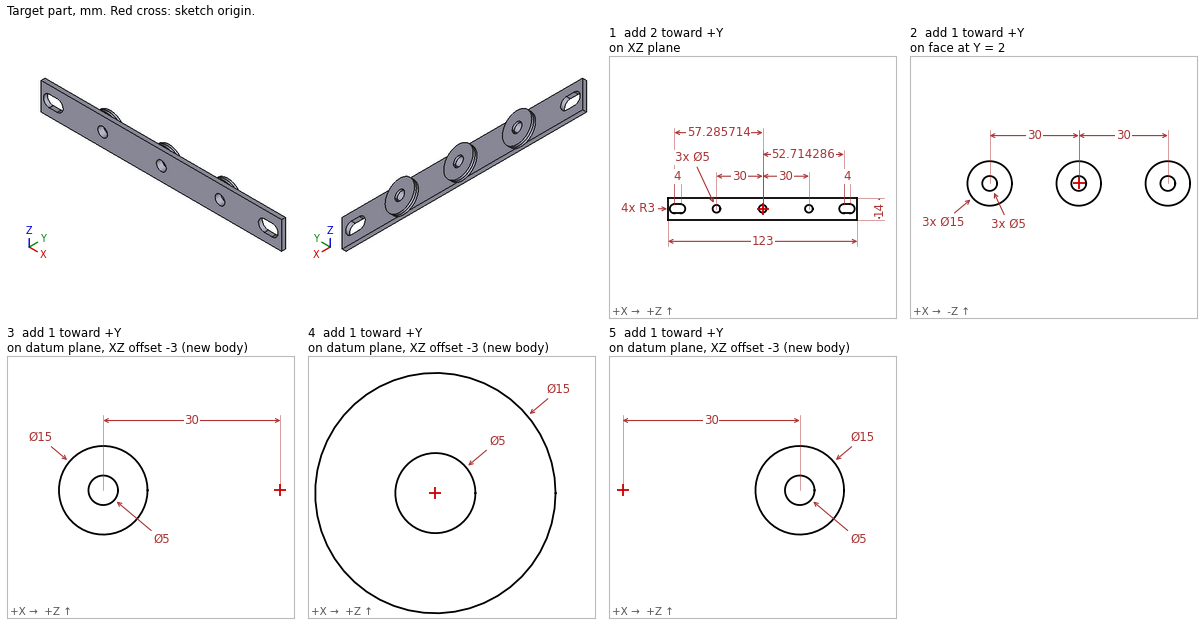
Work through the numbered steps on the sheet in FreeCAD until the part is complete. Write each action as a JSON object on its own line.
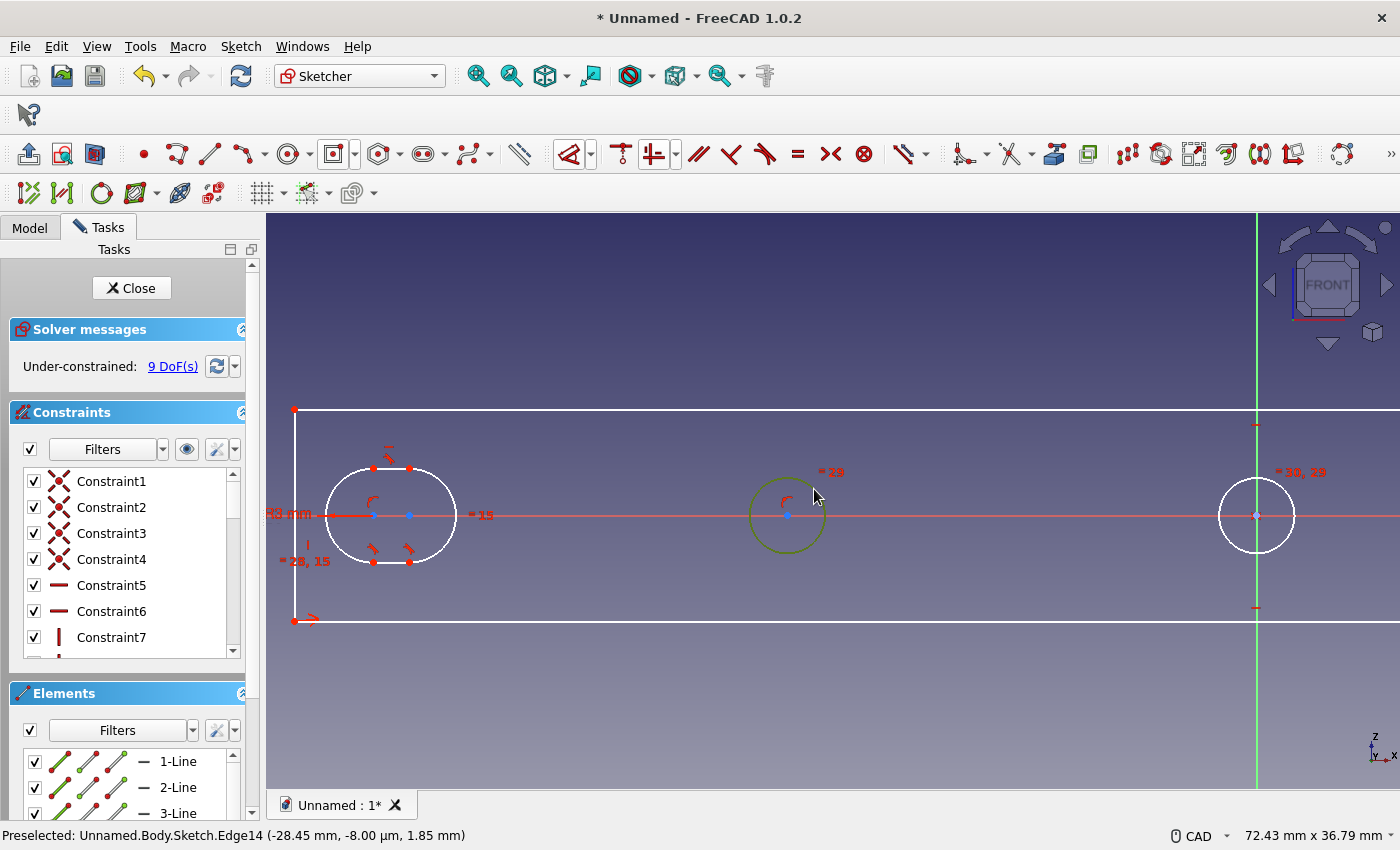
{"action": "left_click", "coordinate": [590, 154]}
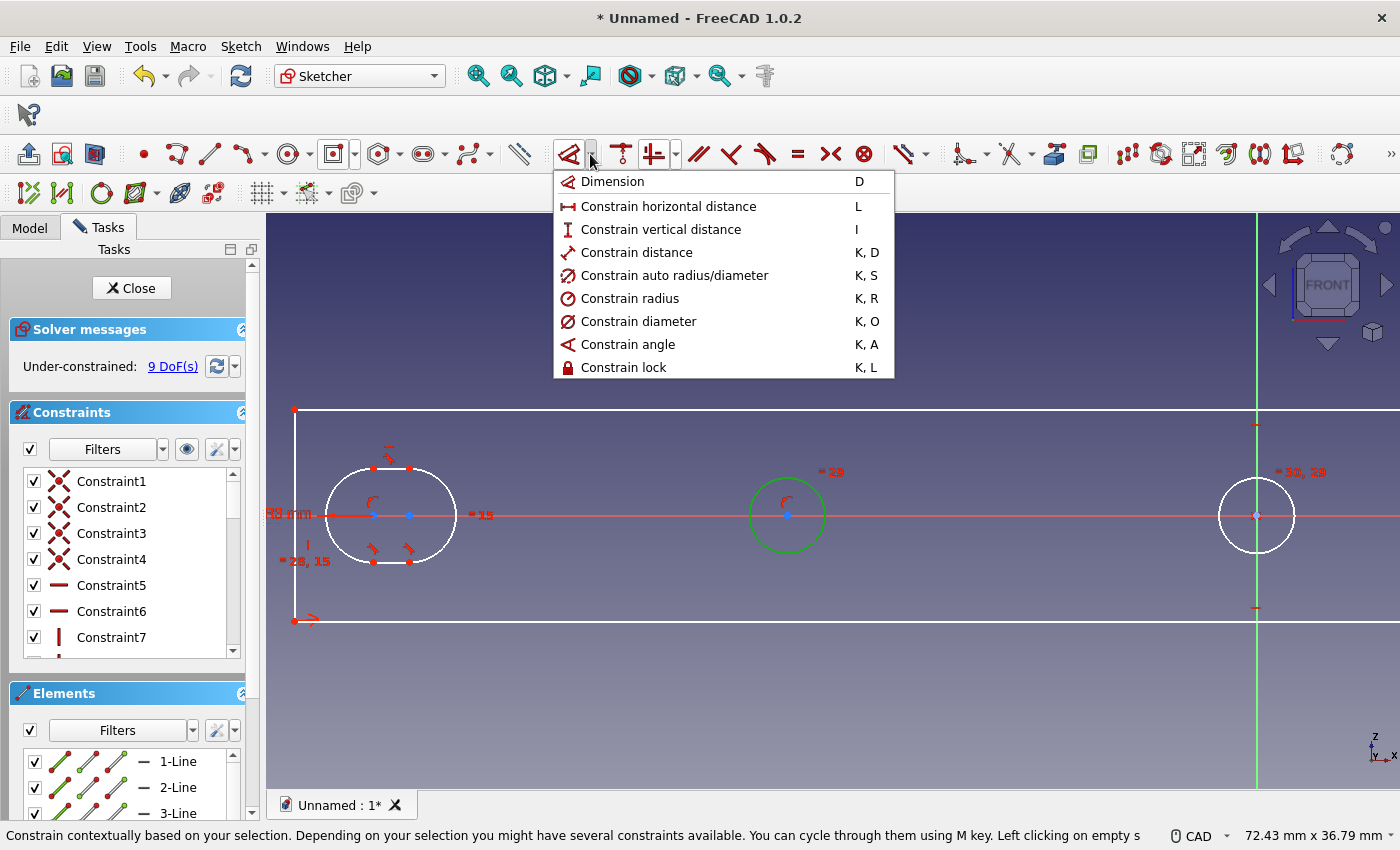
{"action": "left_click", "coordinate": [724, 322]}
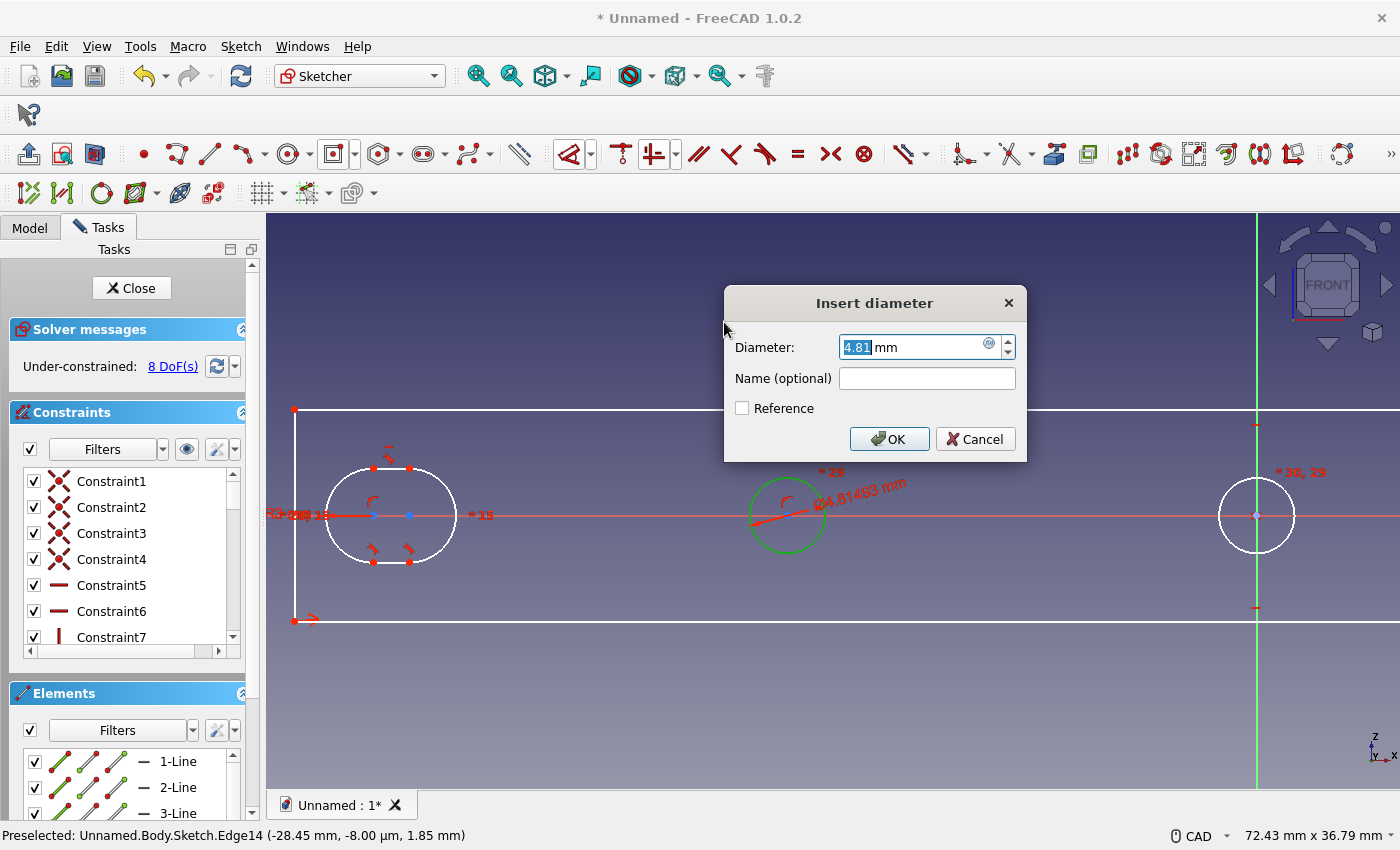
{"action": "type", "text": "5"}
{"action": "key", "text": "Return"}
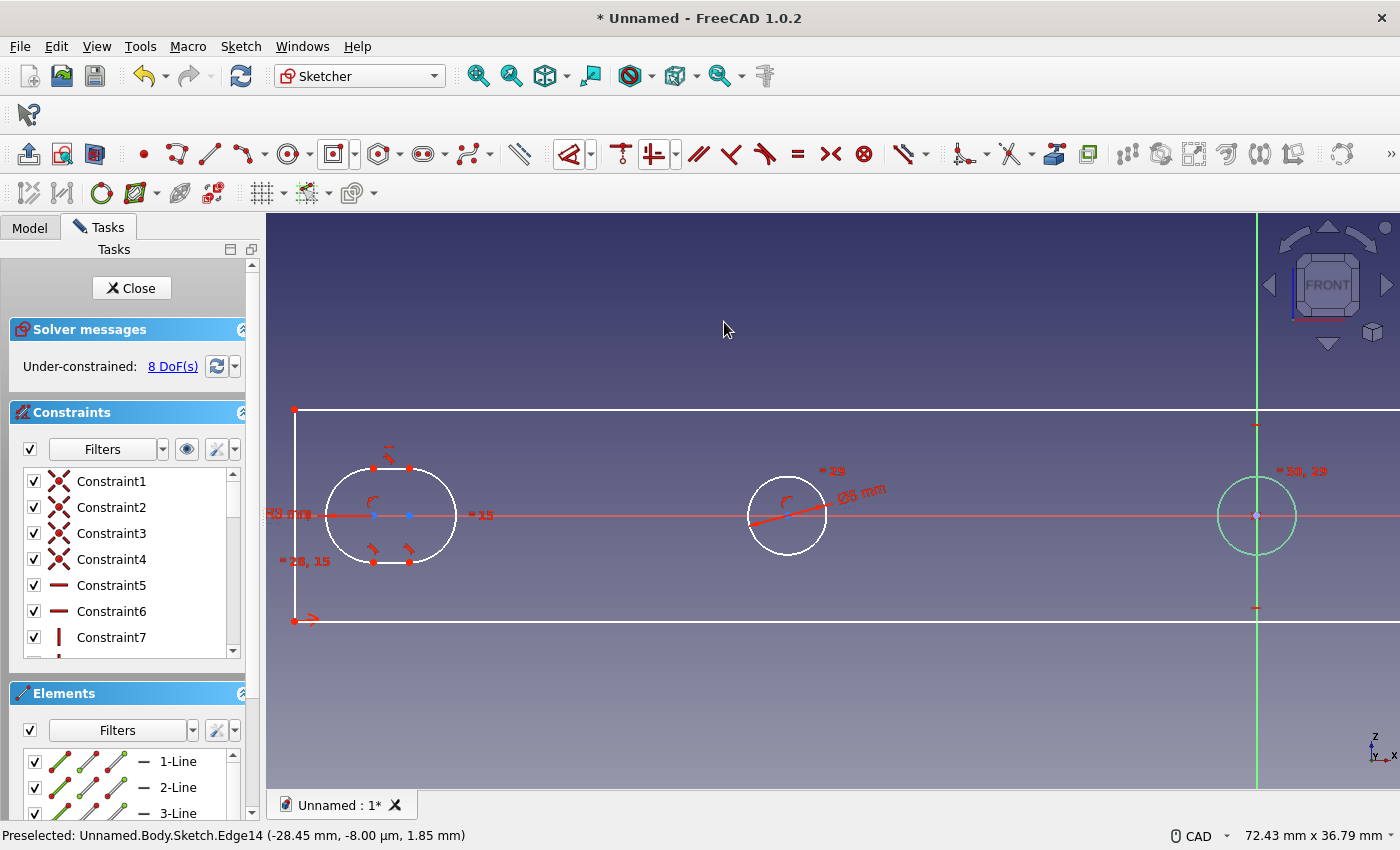
{"action": "scroll", "coordinate": [384, 469], "scroll_direction": "up", "scroll_amount": 2}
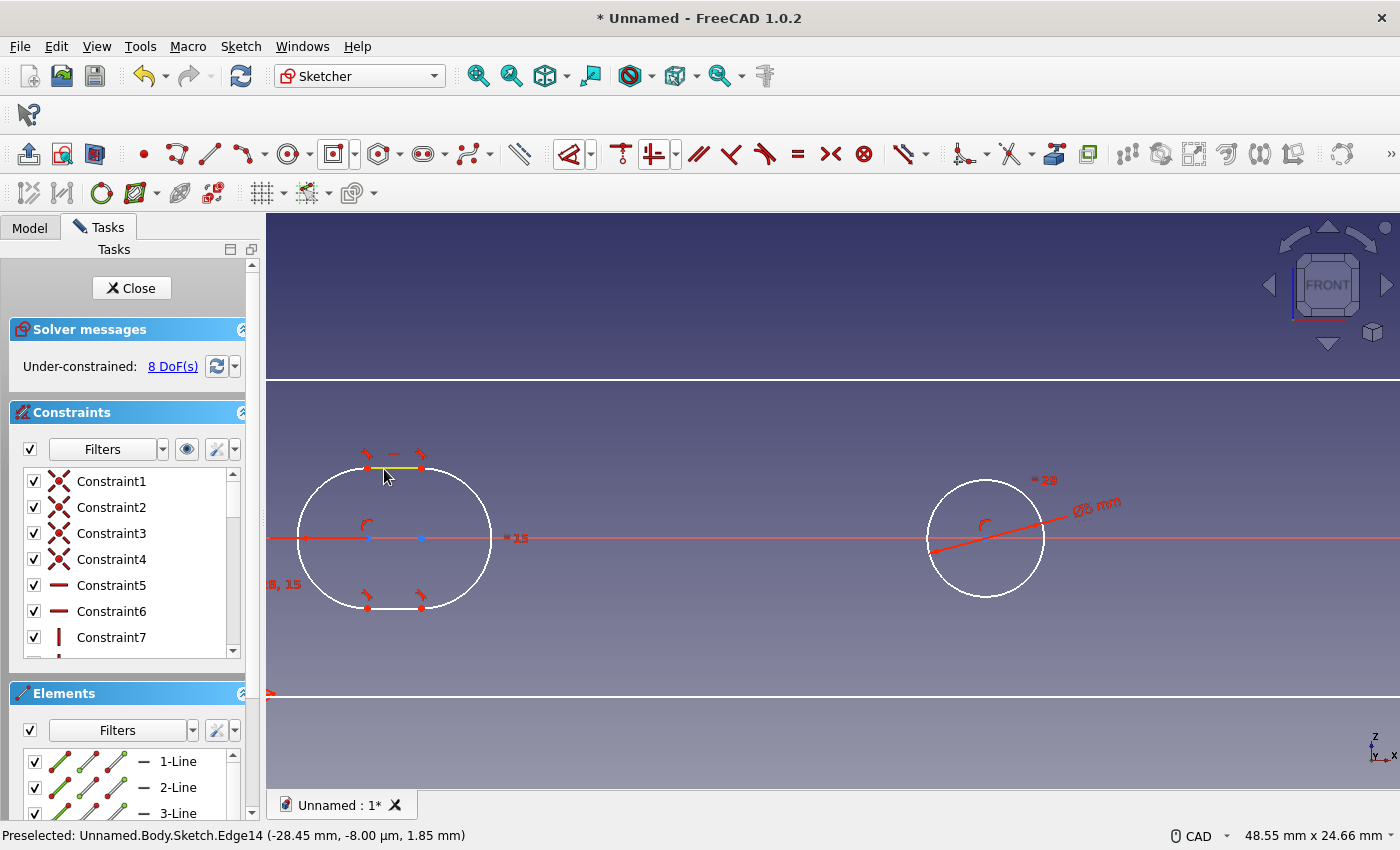
{"action": "left_click", "coordinate": [384, 468]}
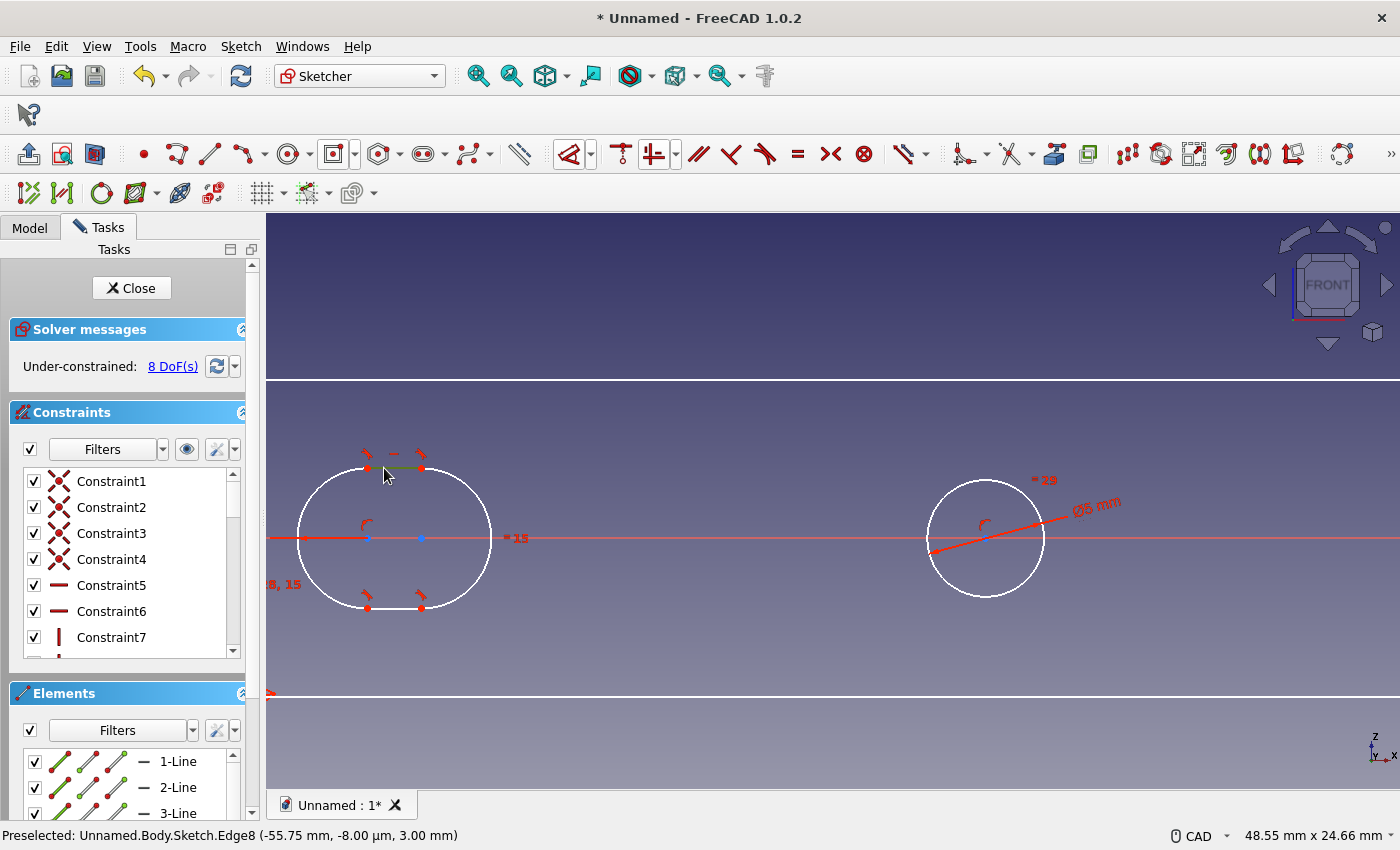
{"action": "key", "text": "l"}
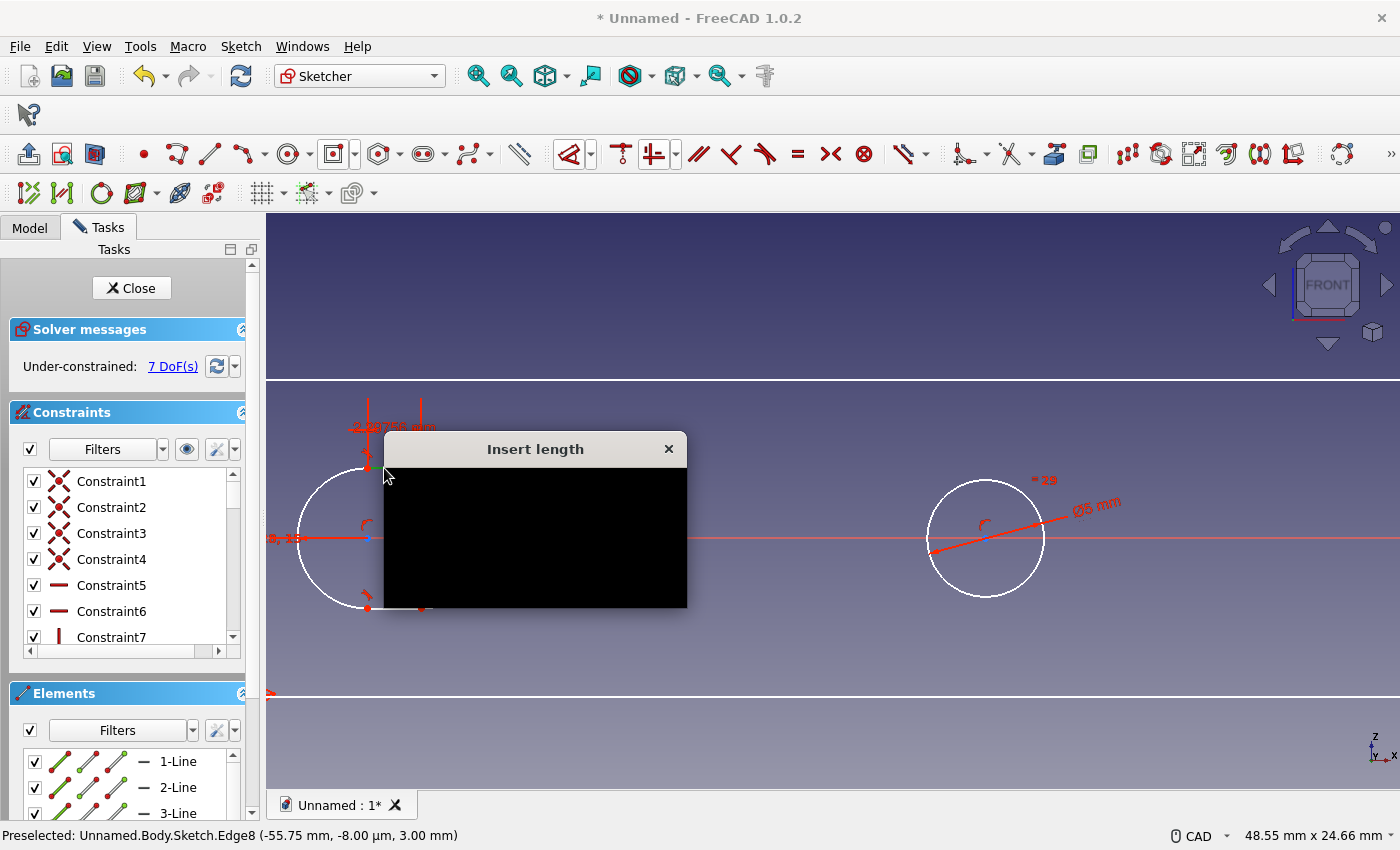
{"action": "type", "text": "4"}
{"action": "key", "text": "Return"}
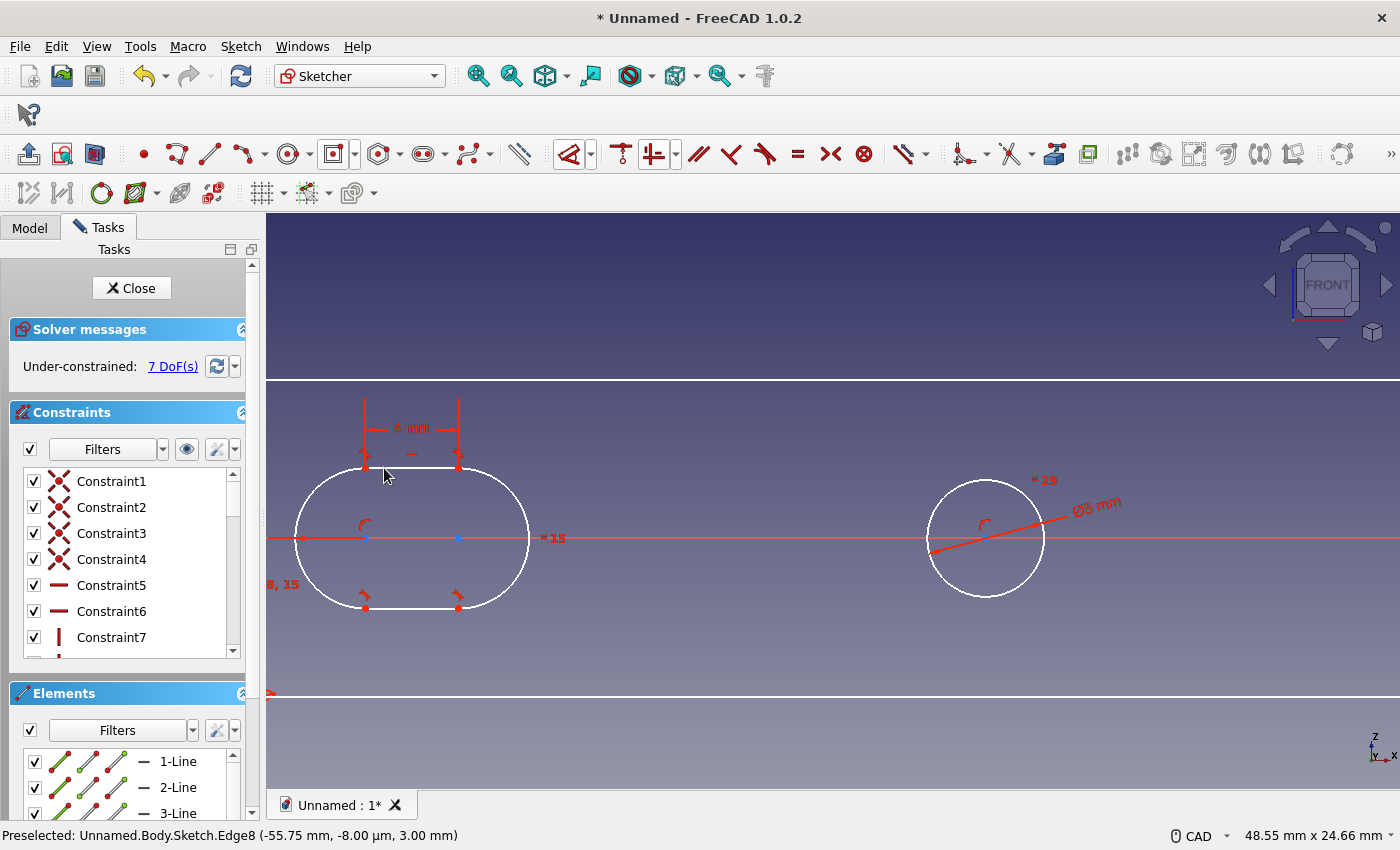
{"action": "scroll", "coordinate": [463, 489], "scroll_direction": "down", "scroll_amount": 7}